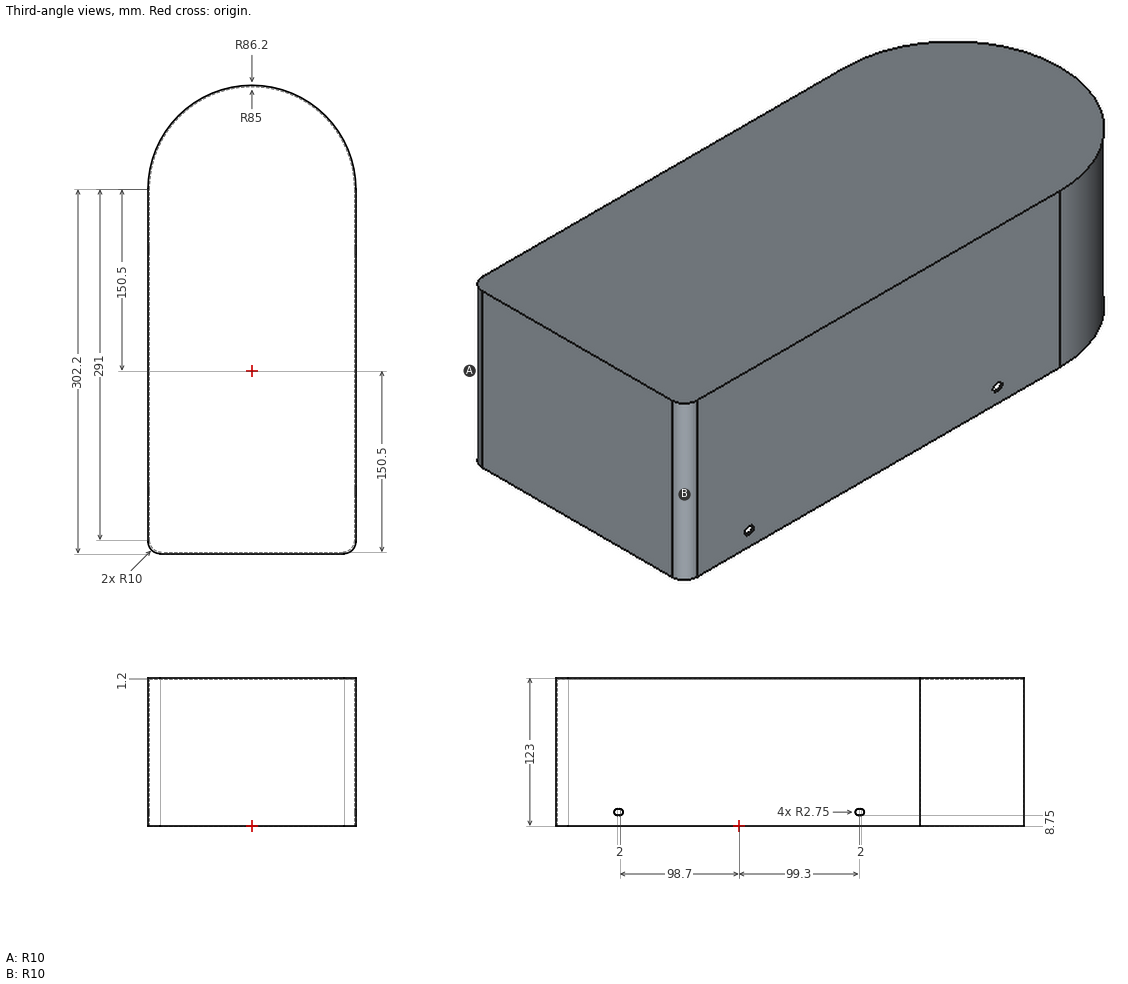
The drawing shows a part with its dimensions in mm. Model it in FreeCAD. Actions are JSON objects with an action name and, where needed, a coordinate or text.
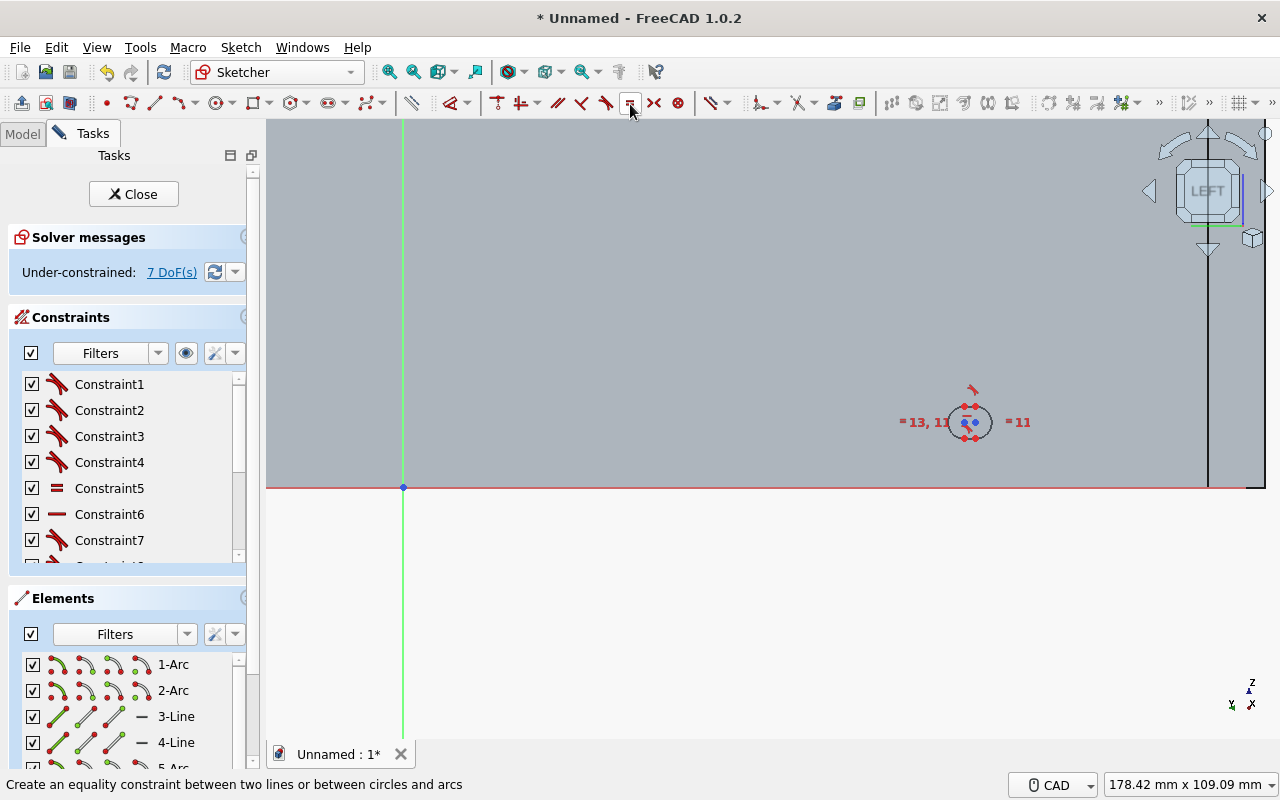
{"action": "left_click", "coordinate": [450, 104]}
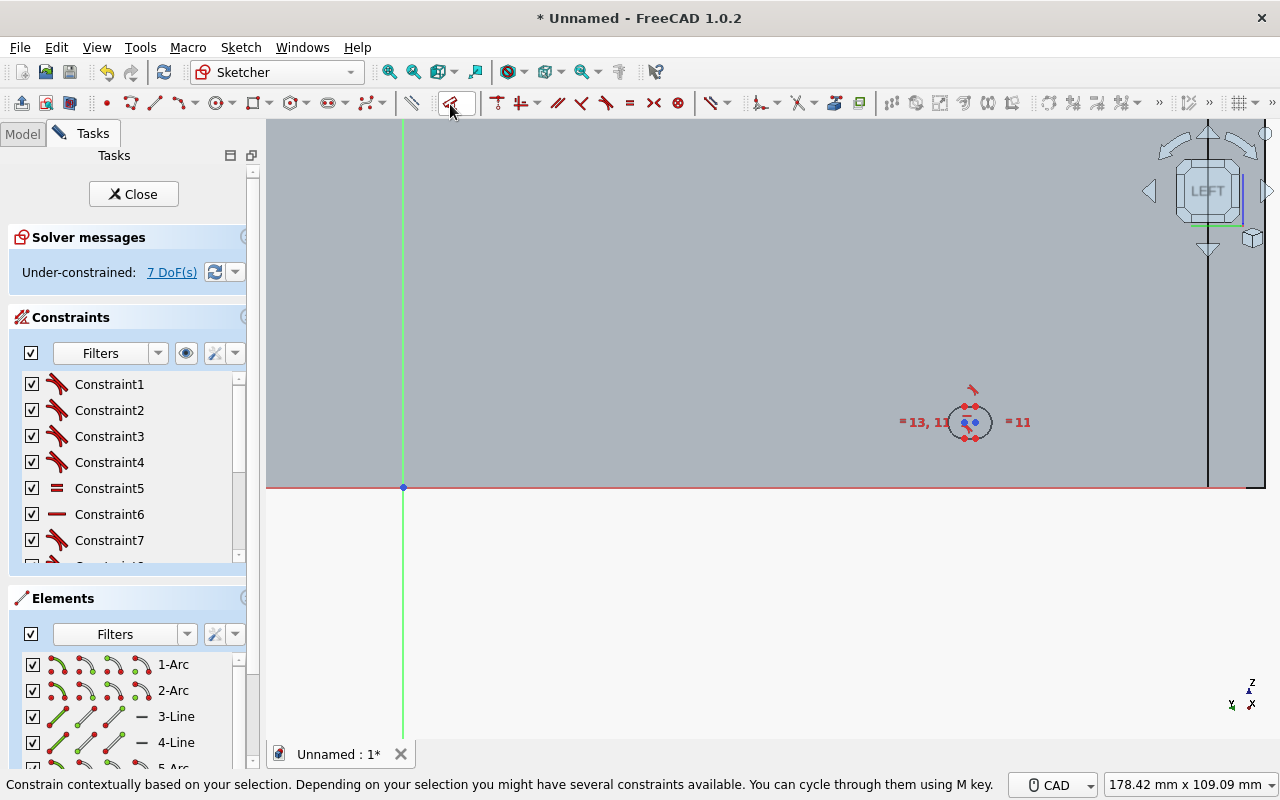
{"action": "scroll", "coordinate": [952, 414], "scroll_direction": "down", "scroll_amount": 4}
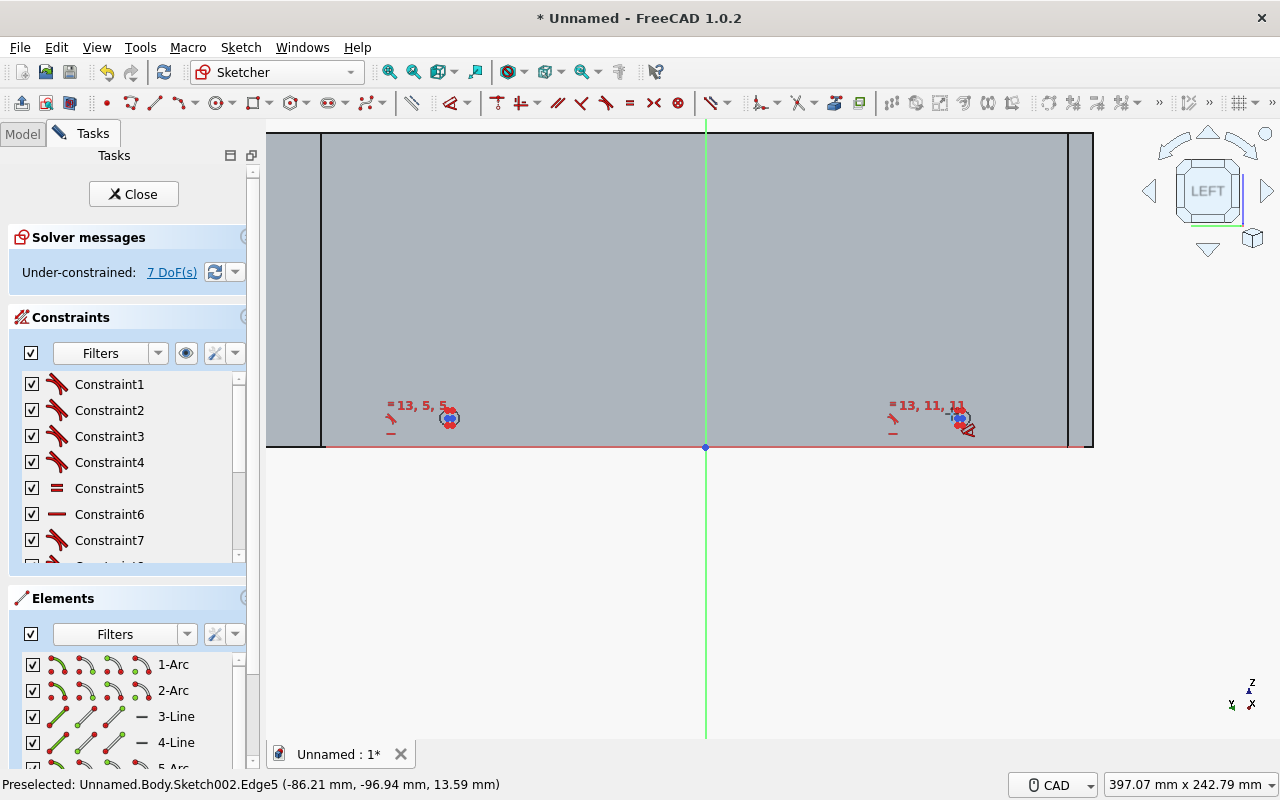
{"action": "scroll", "coordinate": [441, 414], "scroll_direction": "up", "scroll_amount": 9}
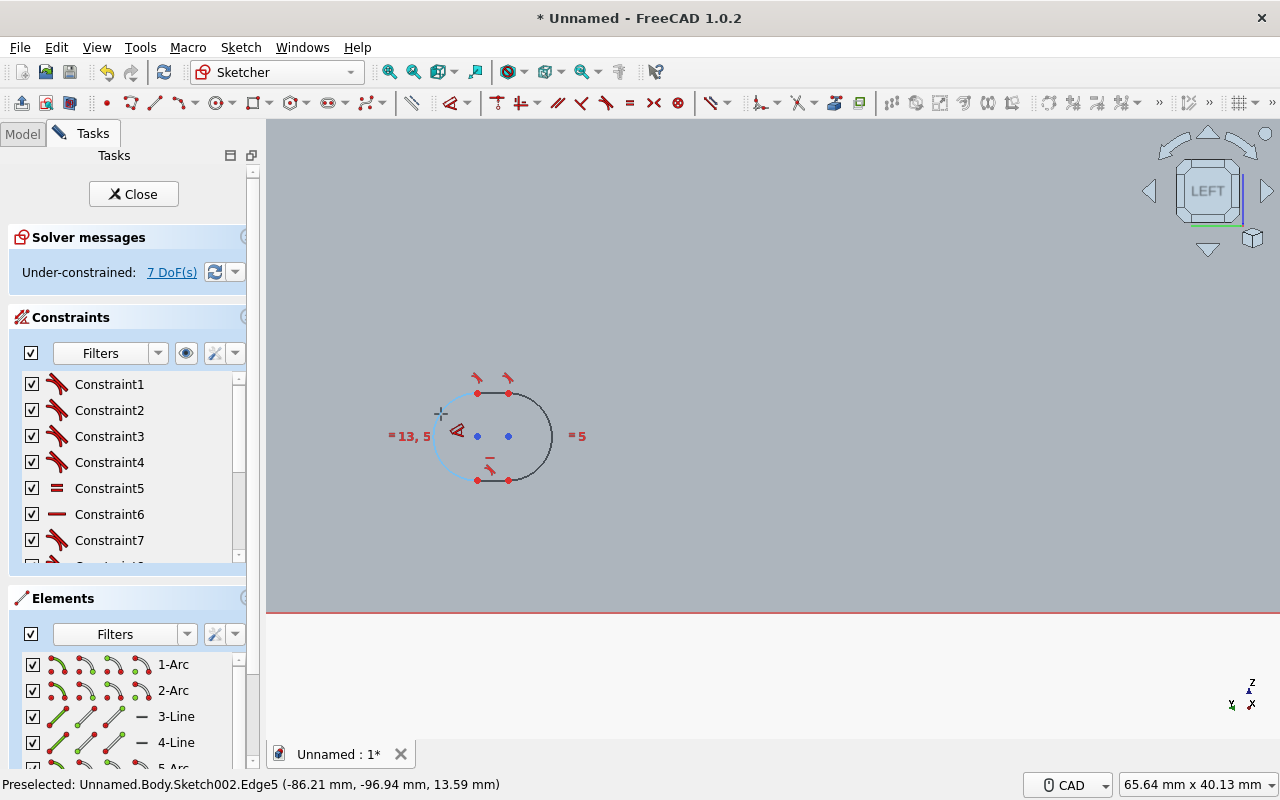
{"action": "left_click", "coordinate": [442, 411]}
{"action": "left_click", "coordinate": [416, 392]}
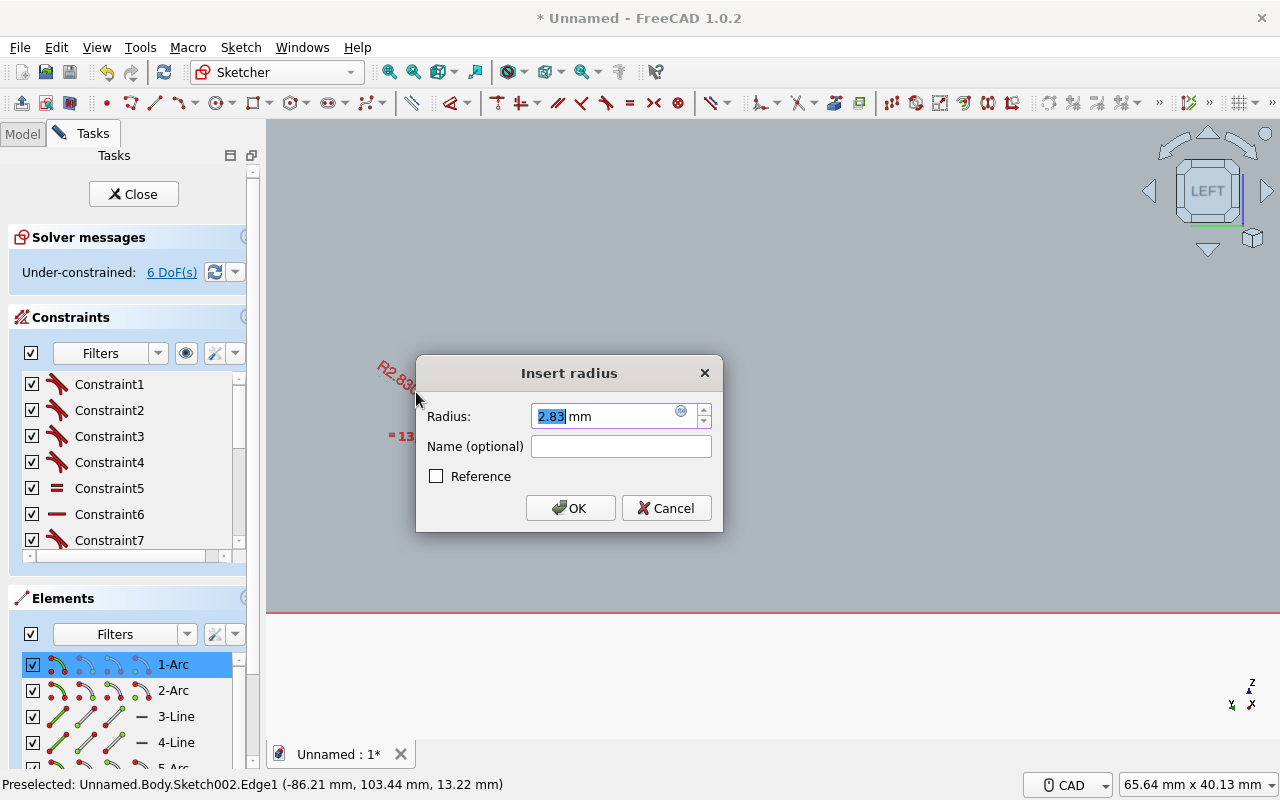
{"action": "type", "text": "2.75"}
{"action": "key", "text": "Return"}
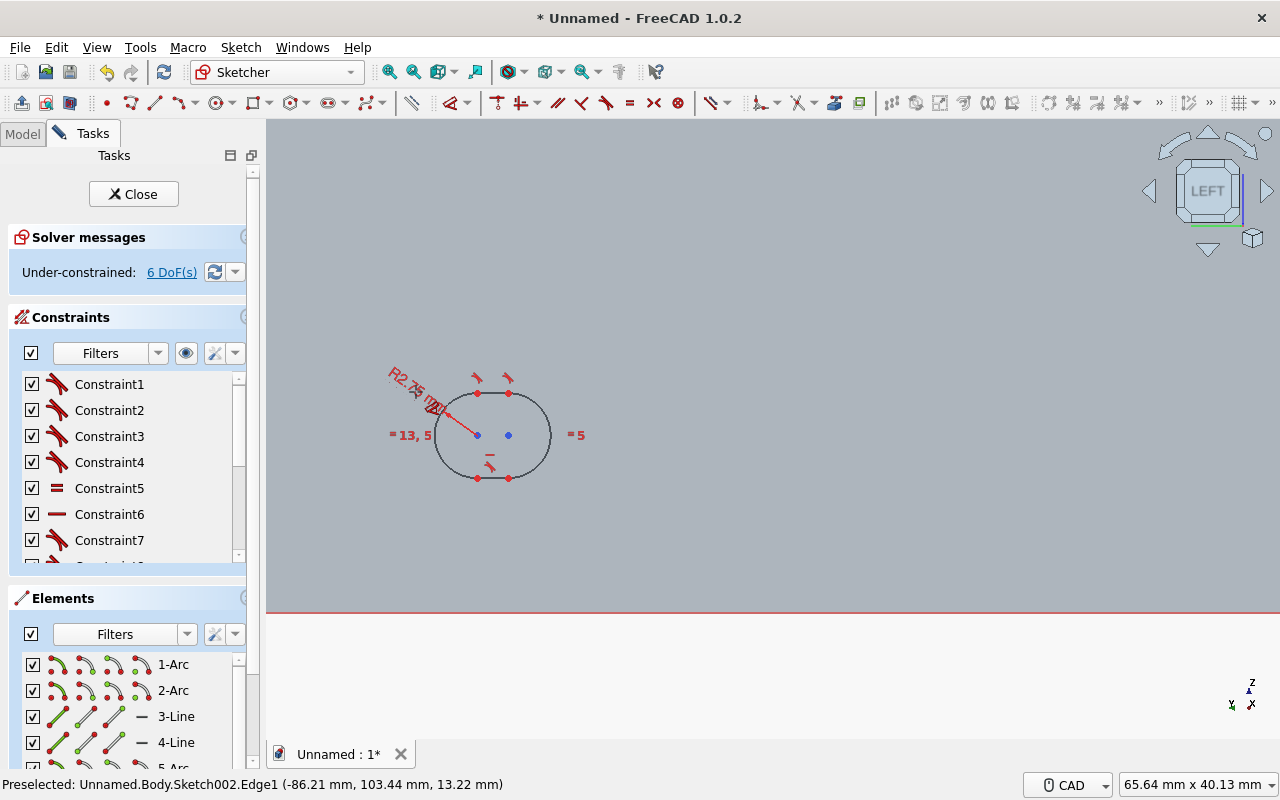
{"action": "scroll", "coordinate": [486, 393], "scroll_direction": "up", "scroll_amount": 2}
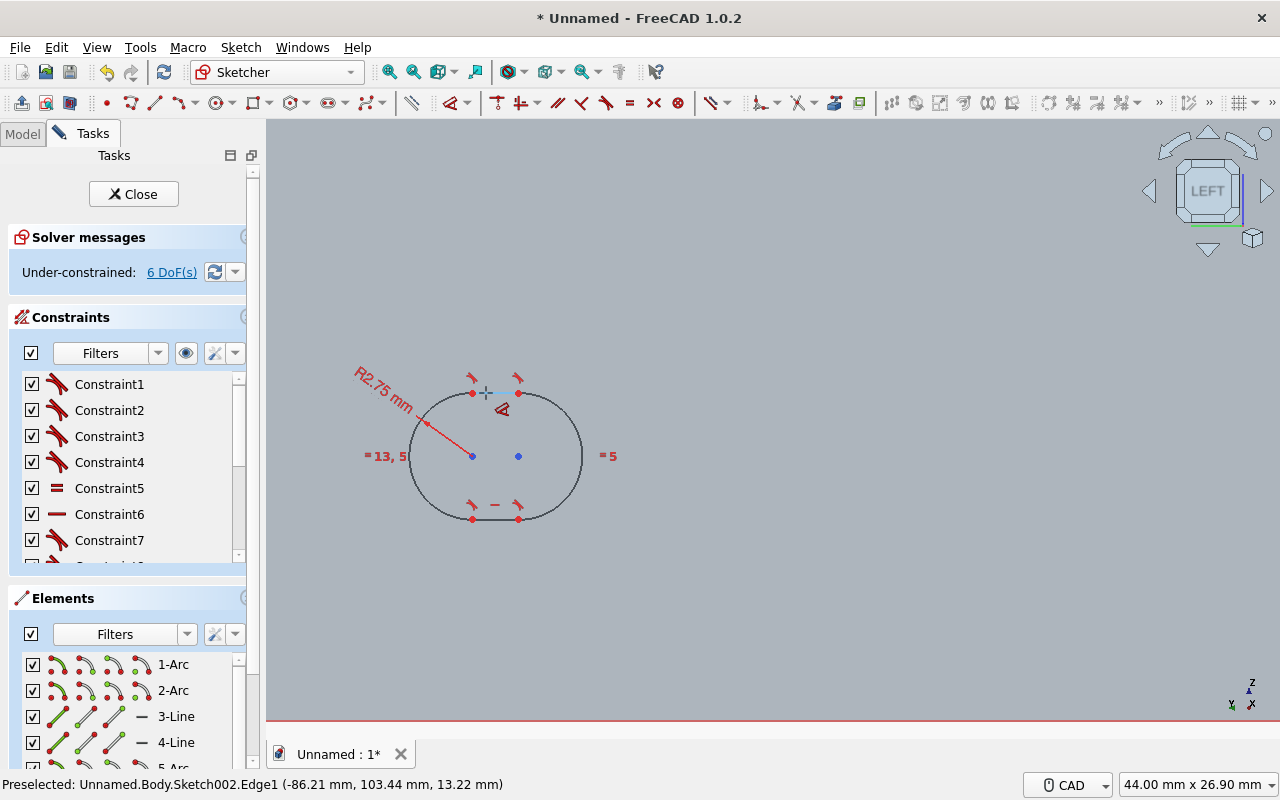
{"action": "left_click", "coordinate": [487, 393]}
{"action": "left_click", "coordinate": [496, 359]}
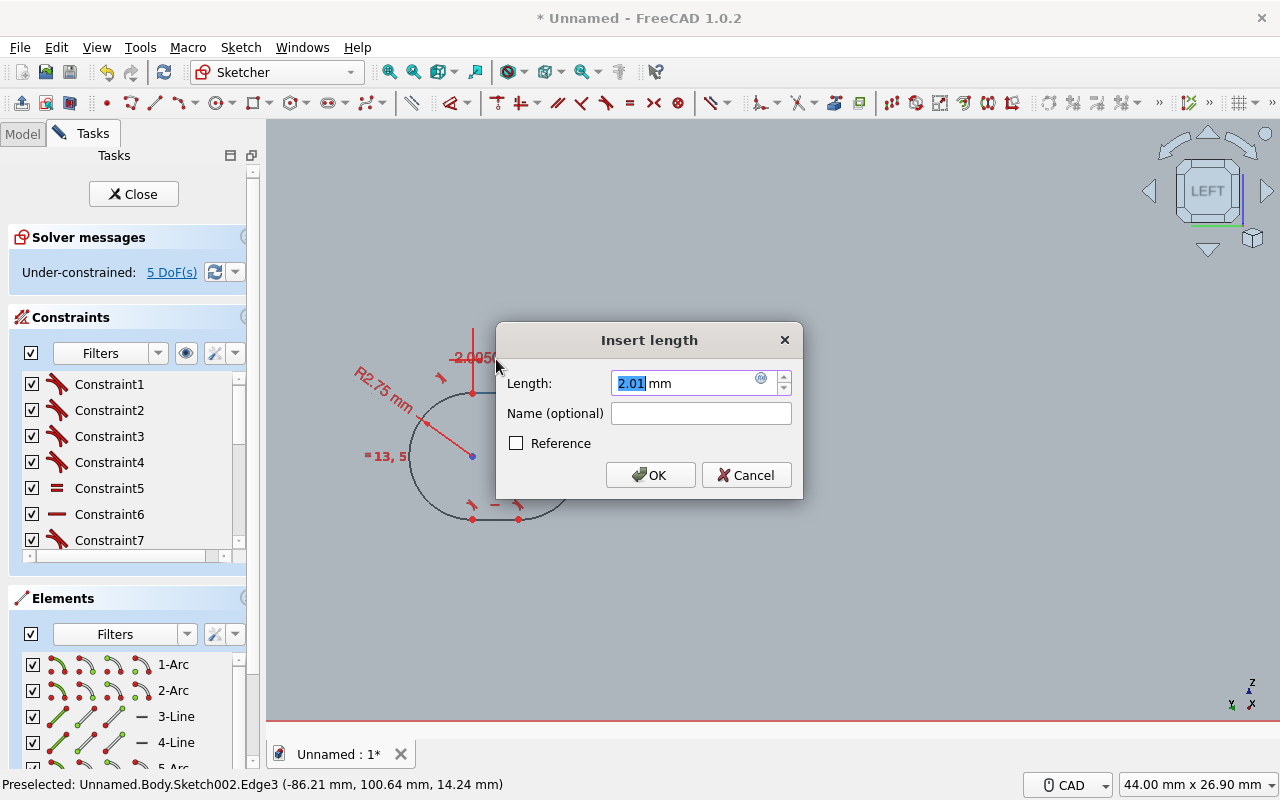
{"action": "type", "text": "2"}
{"action": "key", "text": "Return"}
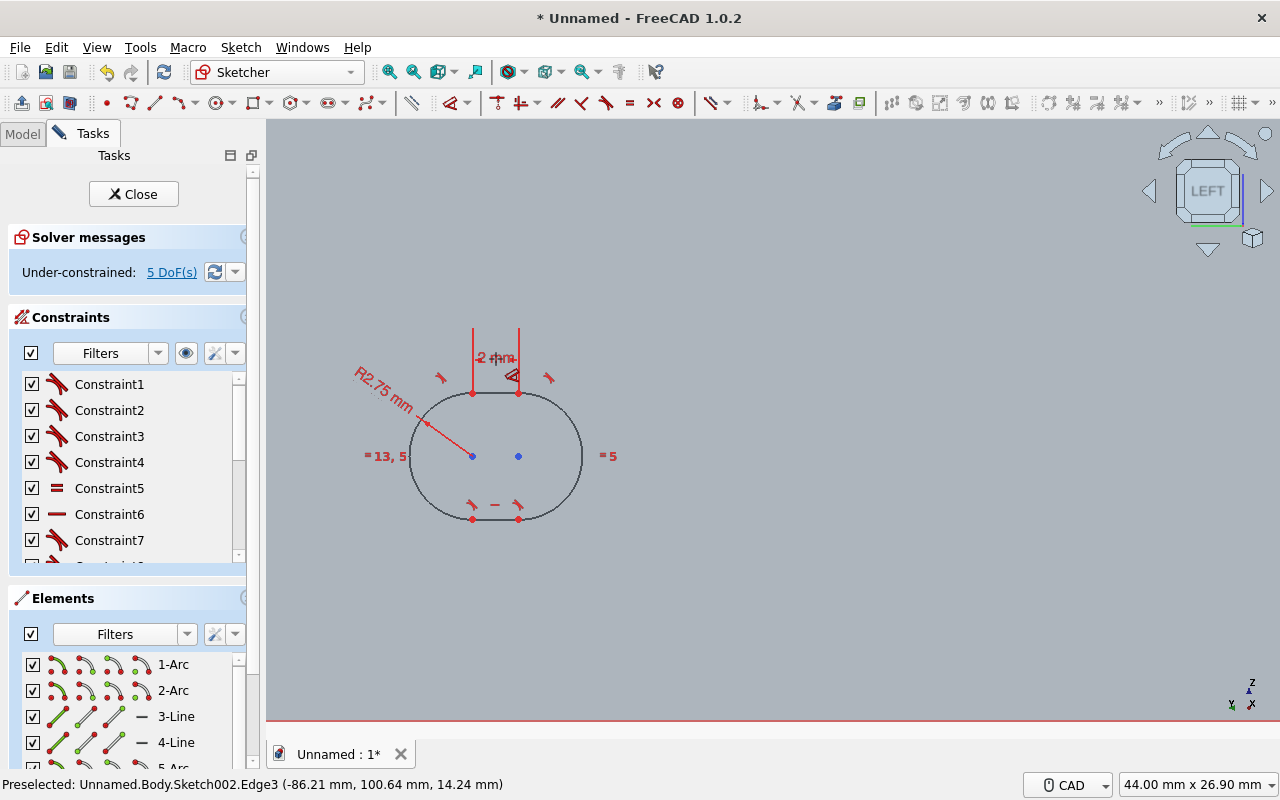
{"action": "scroll", "coordinate": [443, 413], "scroll_direction": "down", "scroll_amount": 11}